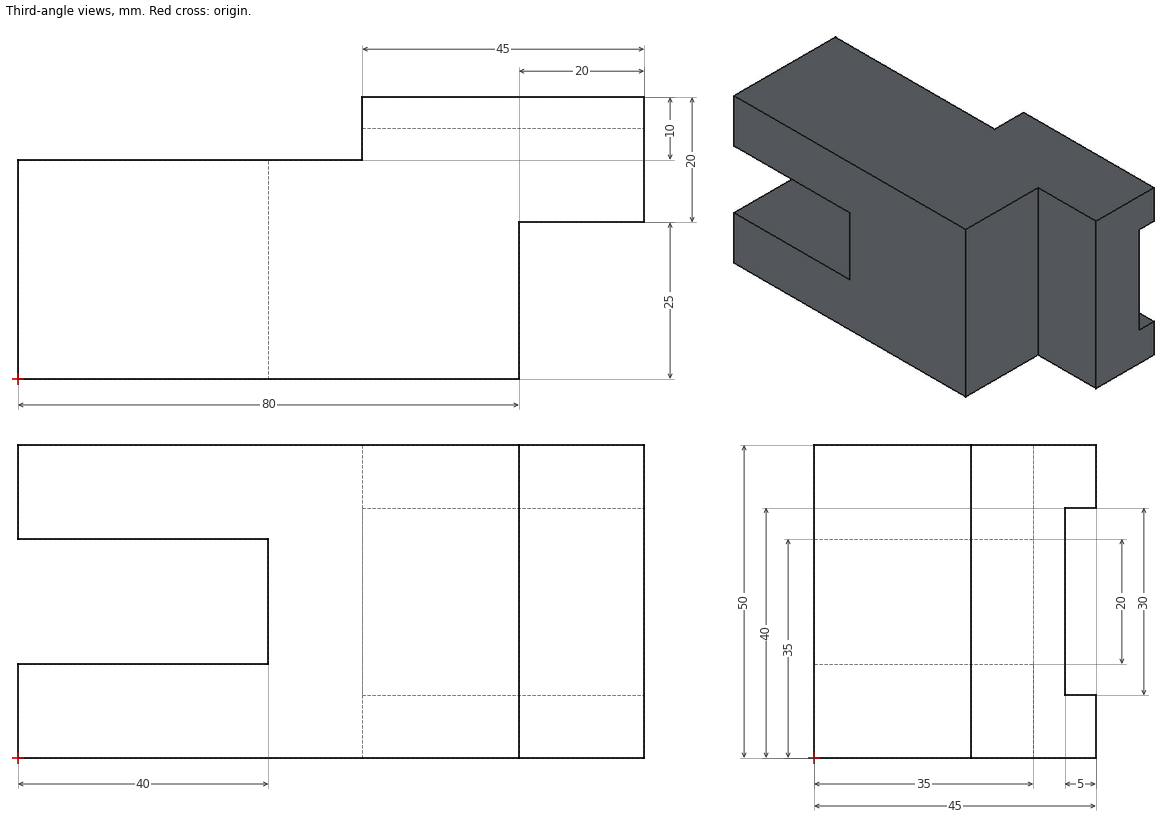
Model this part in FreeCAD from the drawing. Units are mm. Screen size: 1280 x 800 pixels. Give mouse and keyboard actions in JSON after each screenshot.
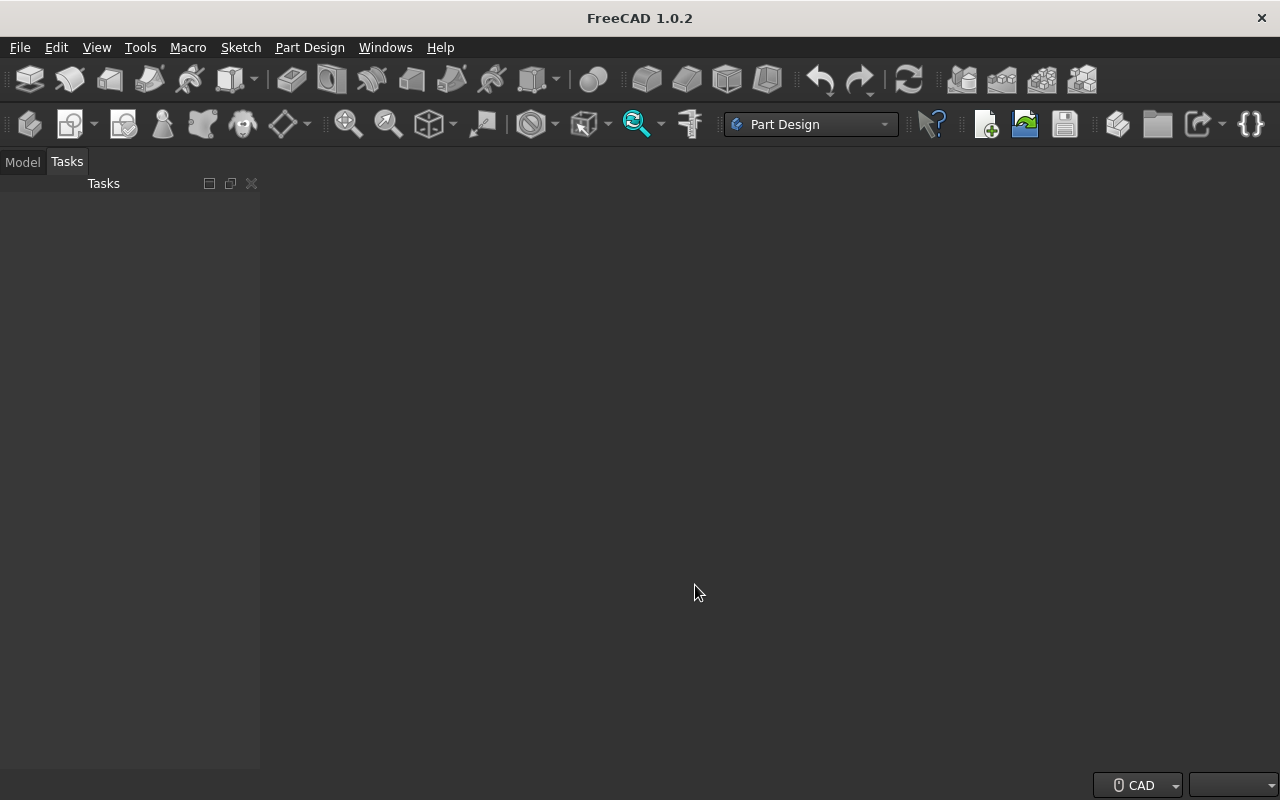
{"action": "left_click", "coordinate": [986, 124]}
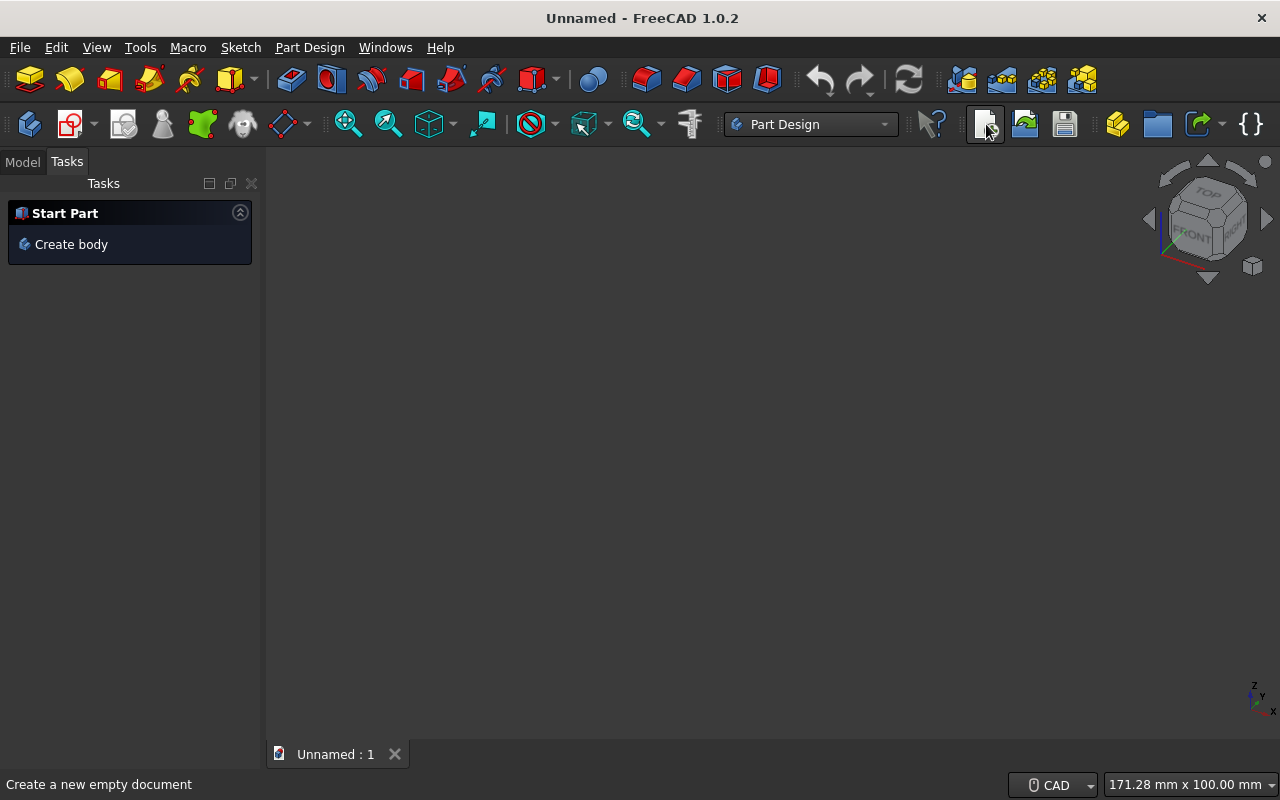
{"action": "left_click", "coordinate": [70, 124]}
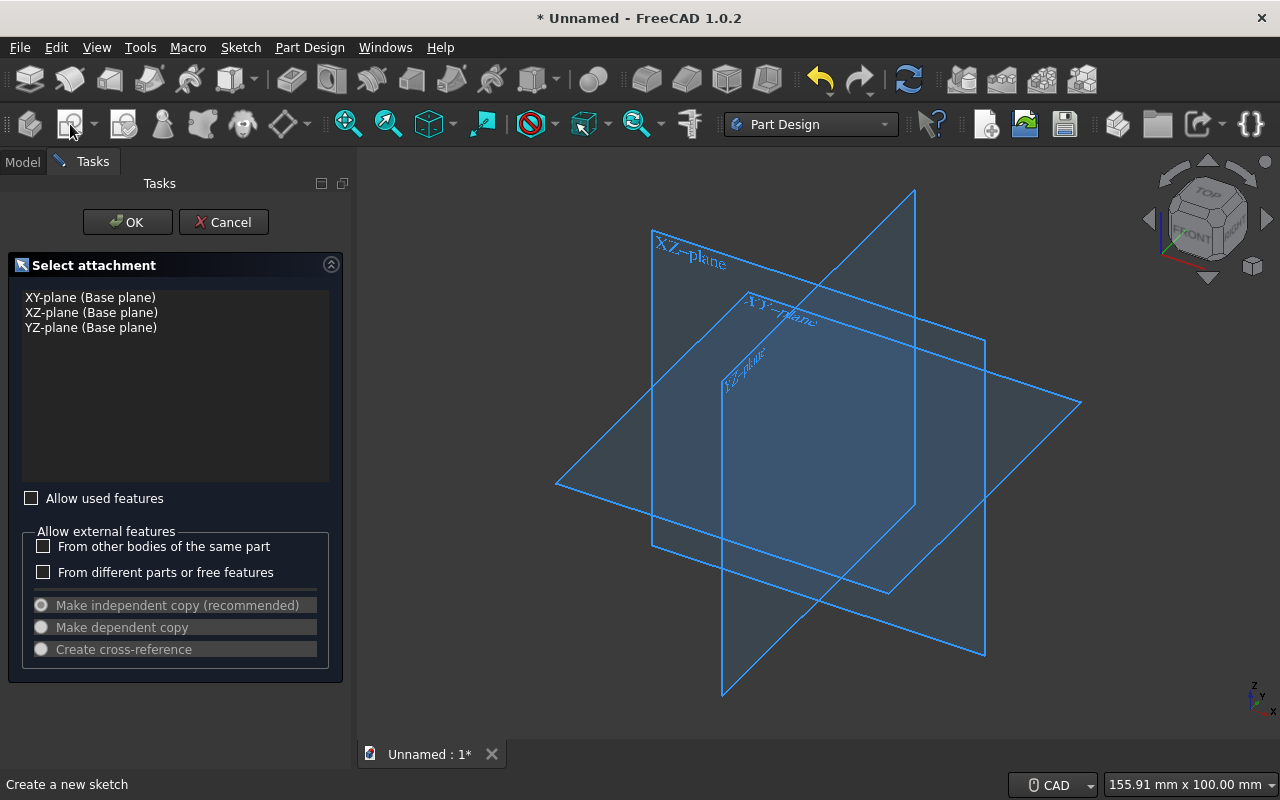
{"action": "left_click", "coordinate": [82, 298]}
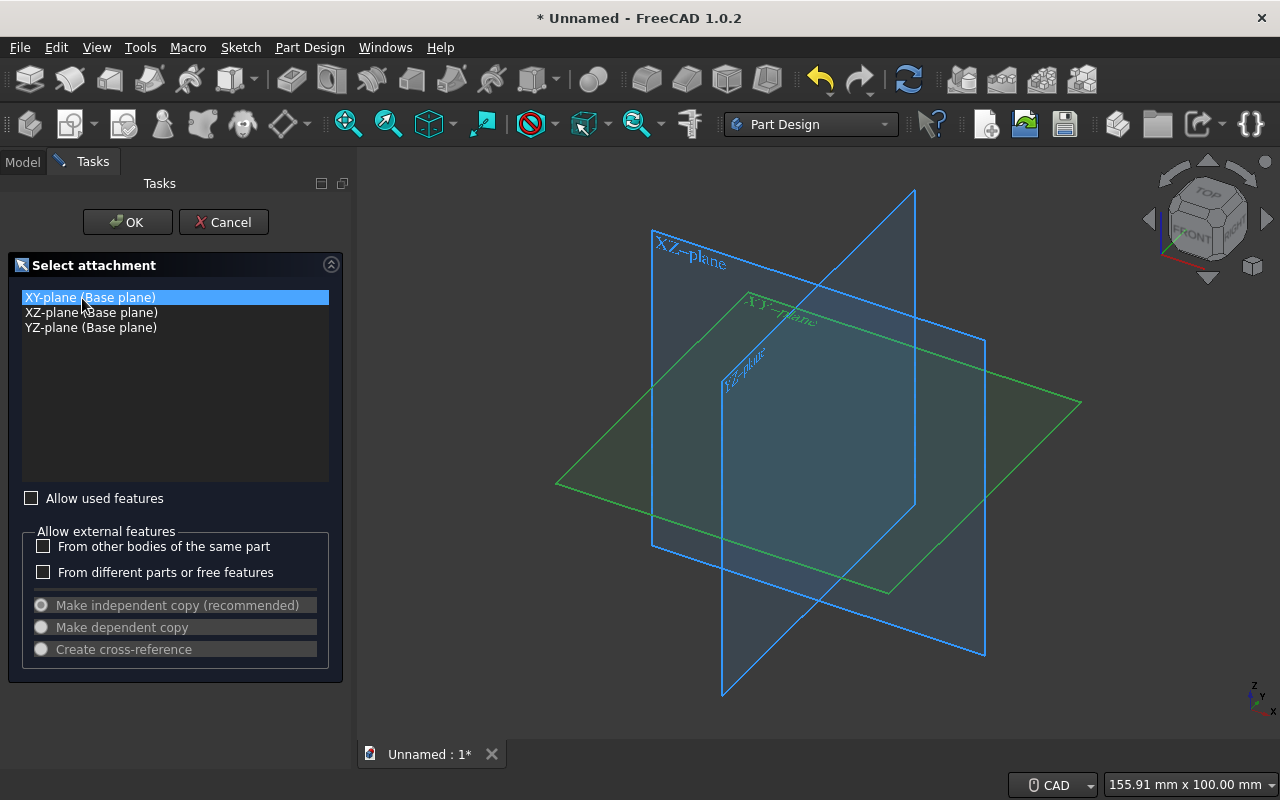
{"action": "left_click", "coordinate": [128, 222]}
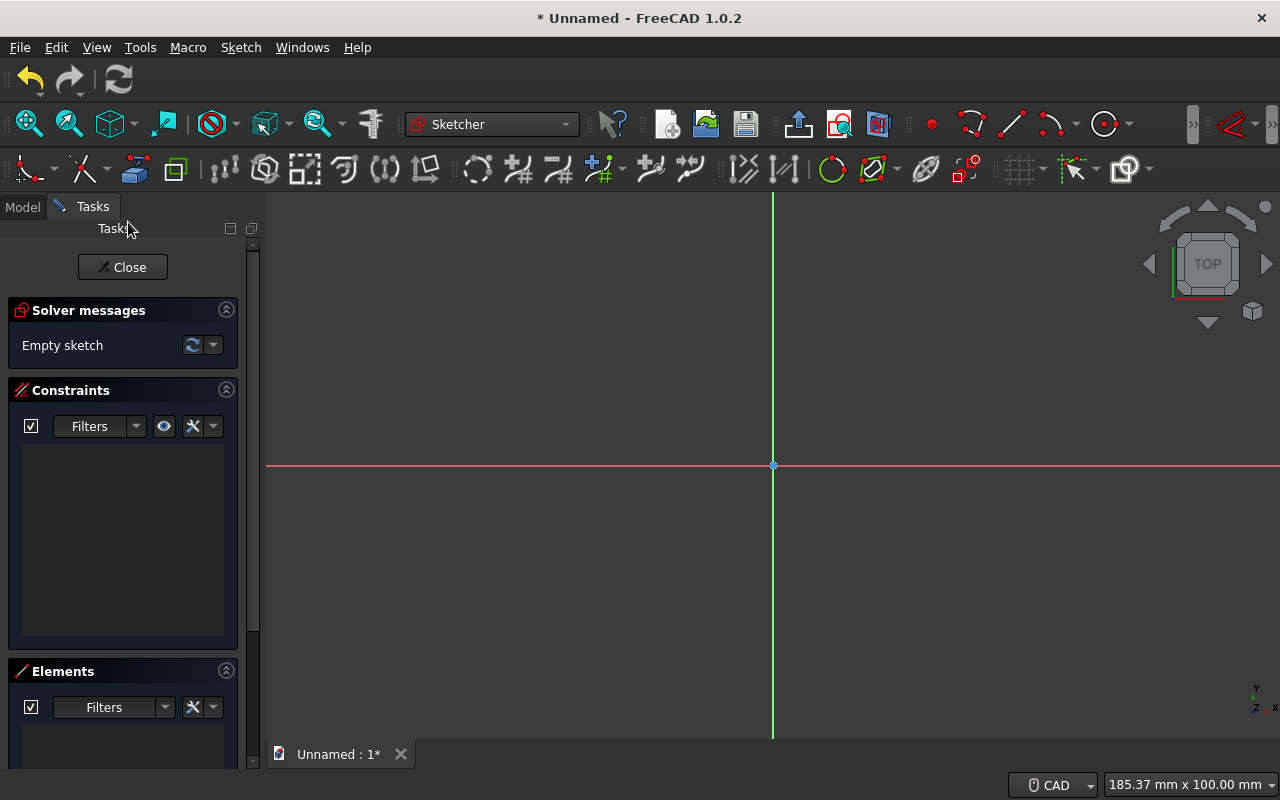
{"action": "scroll", "coordinate": [294, 711], "scroll_direction": "down", "scroll_amount": 2}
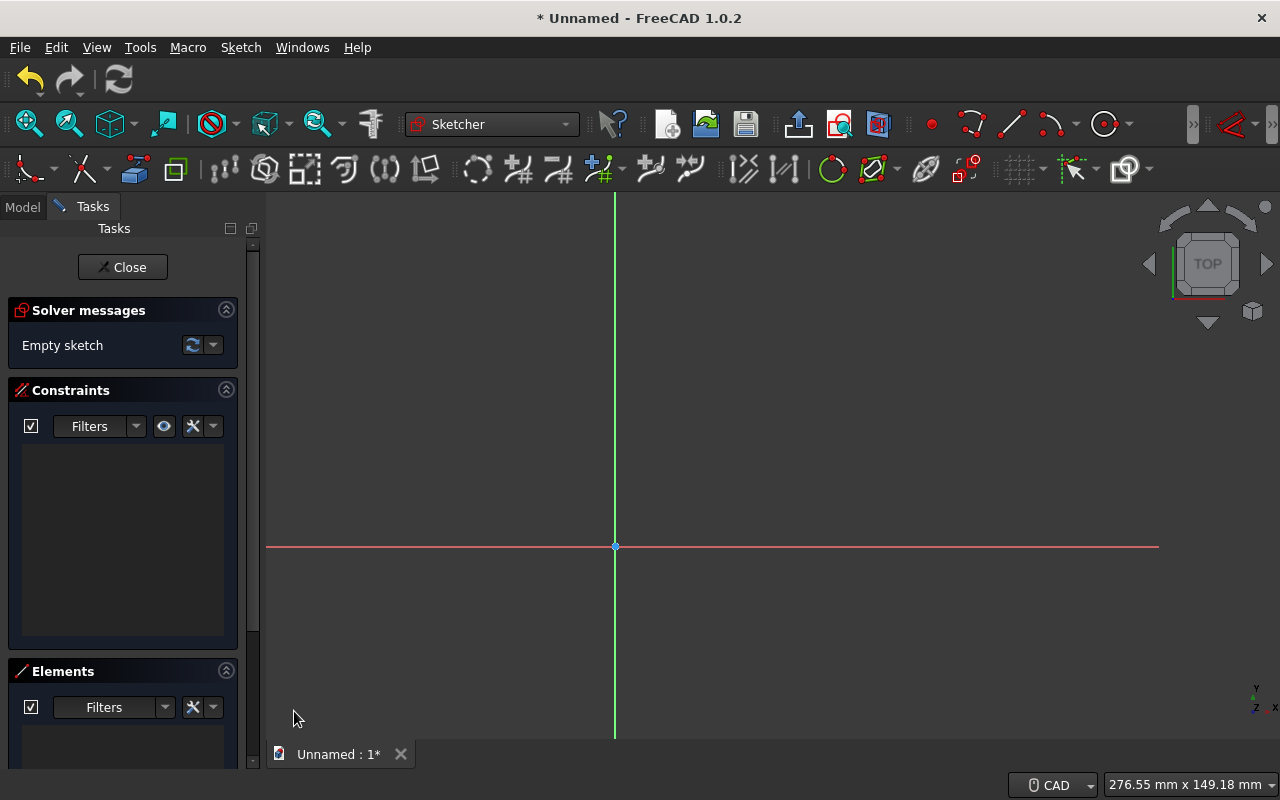
{"action": "scroll", "coordinate": [989, 462], "scroll_direction": "up", "scroll_amount": 2}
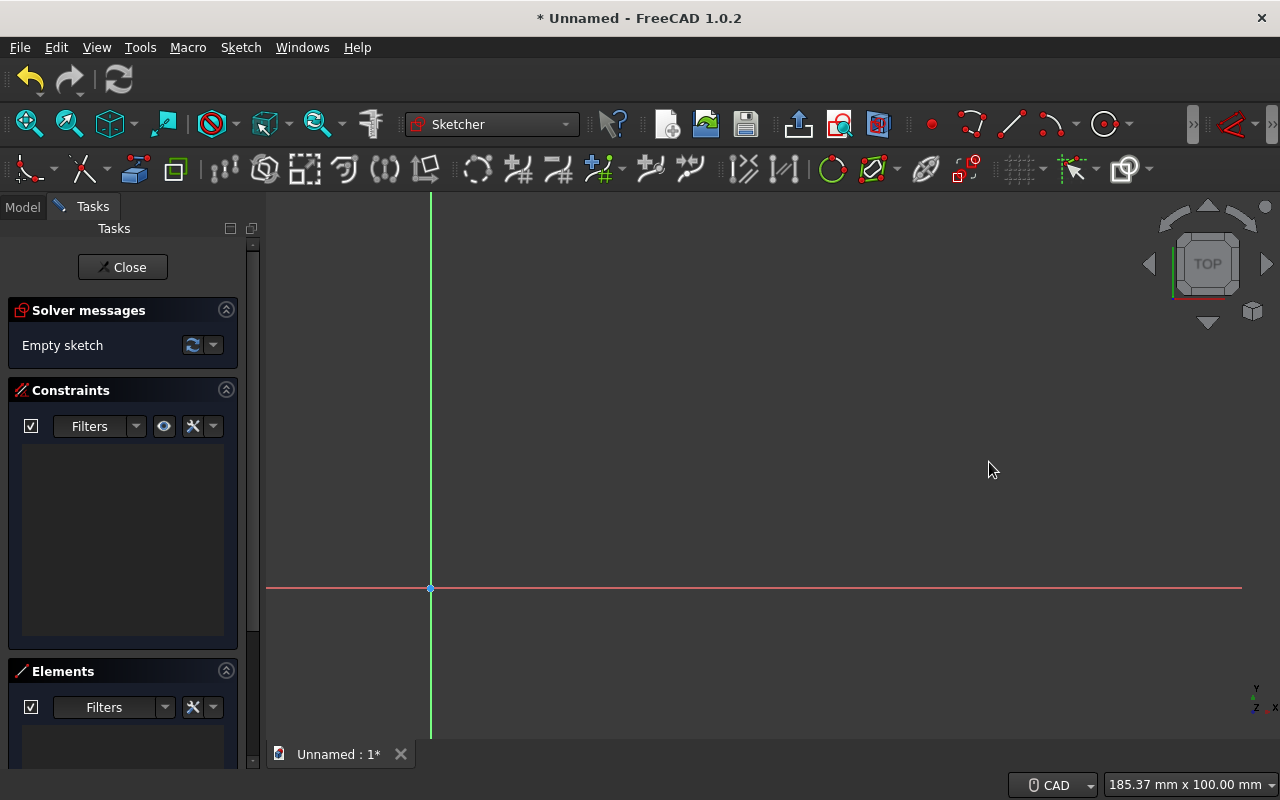
{"action": "key", "text": "g m"}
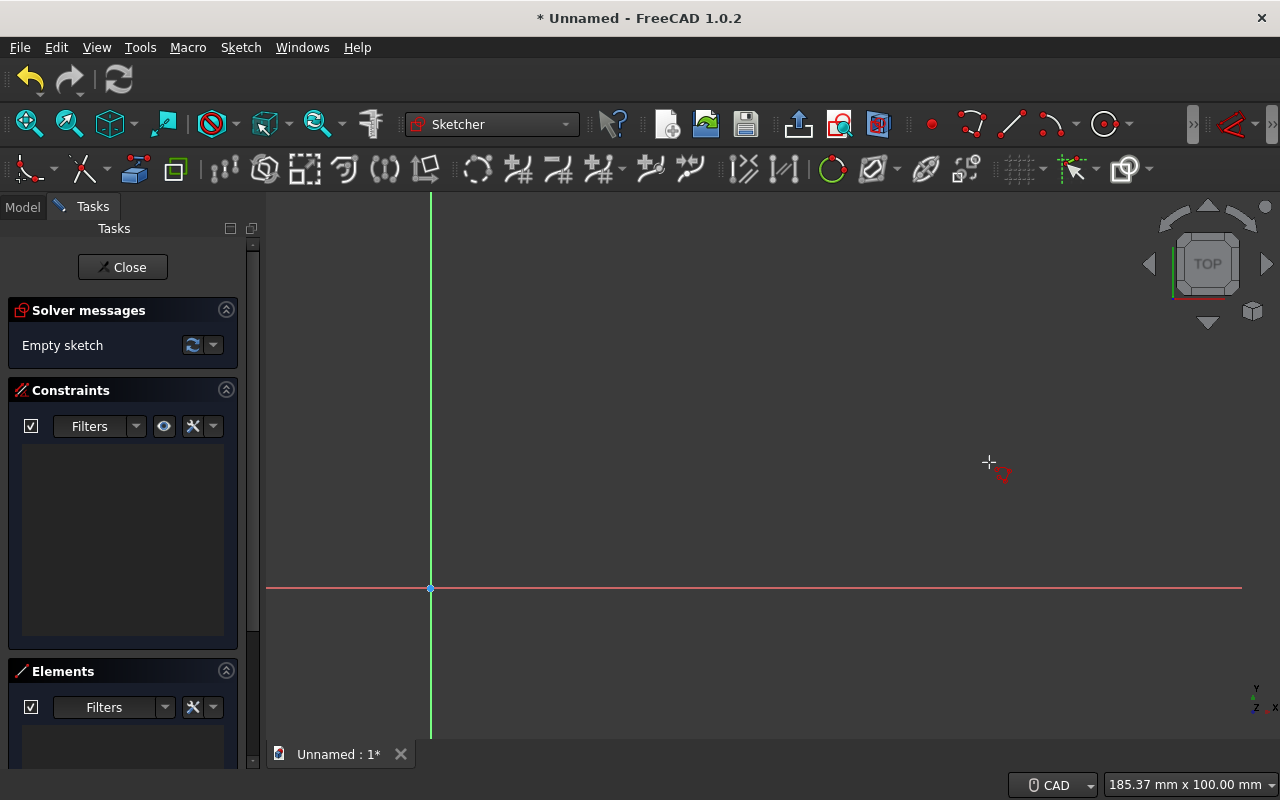
{"action": "left_click", "coordinate": [431, 588]}
{"action": "left_click", "coordinate": [868, 579]}
{"action": "left_click", "coordinate": [868, 451]}
{"action": "left_click", "coordinate": [978, 451]}
{"action": "left_click", "coordinate": [978, 342]}
{"action": "left_click", "coordinate": [732, 342]}
{"action": "left_click", "coordinate": [732, 397]}
{"action": "left_click", "coordinate": [440, 397]}
{"action": "left_click", "coordinate": [431, 588]}
{"action": "key", "text": "Escape"}
{"action": "key", "text": "Escape"}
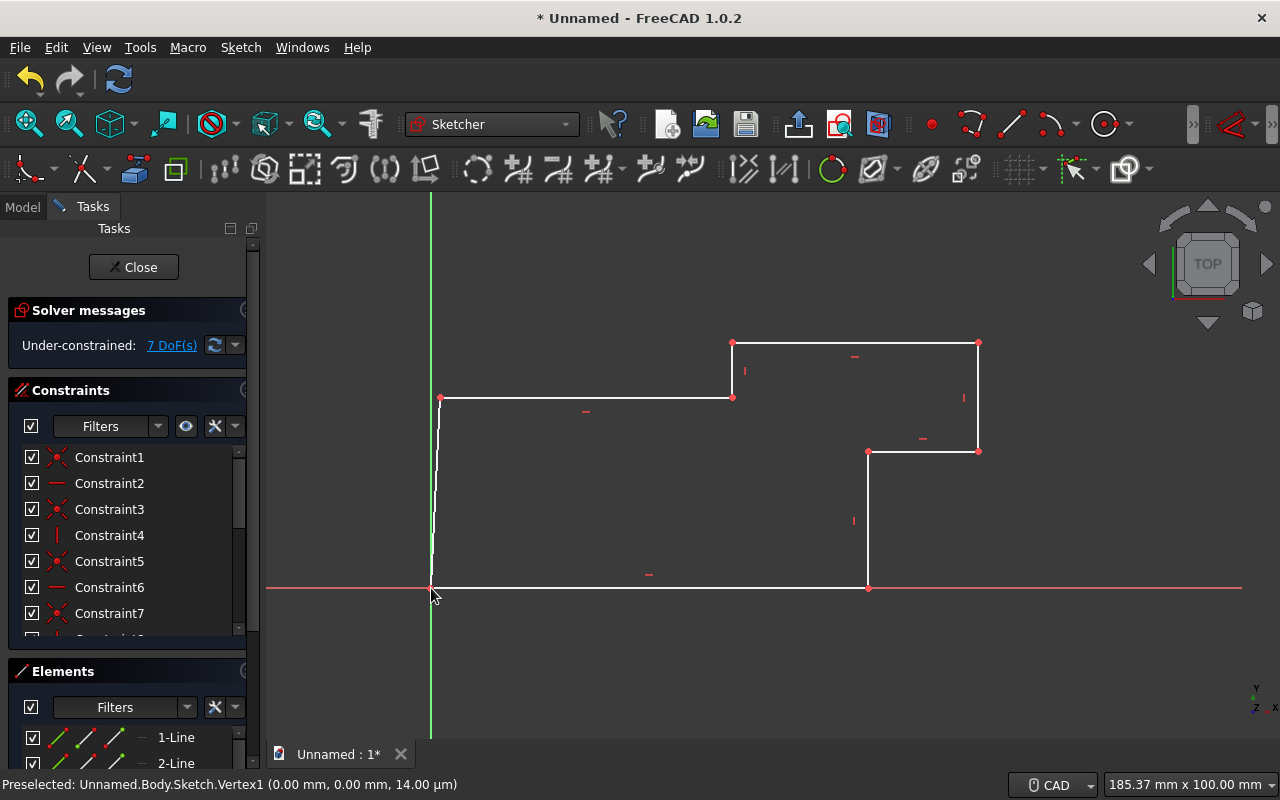
{"action": "left_click", "coordinate": [434, 531]}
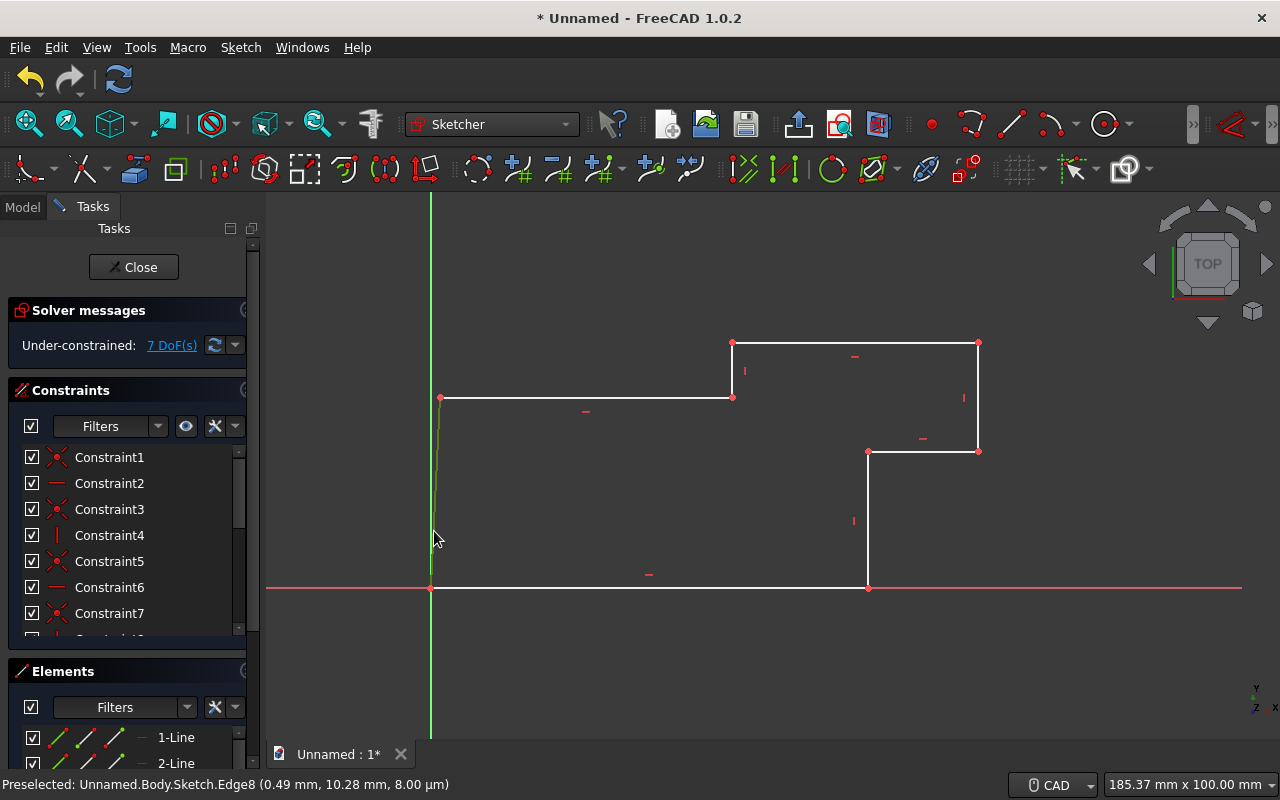
{"action": "key", "text": "v"}